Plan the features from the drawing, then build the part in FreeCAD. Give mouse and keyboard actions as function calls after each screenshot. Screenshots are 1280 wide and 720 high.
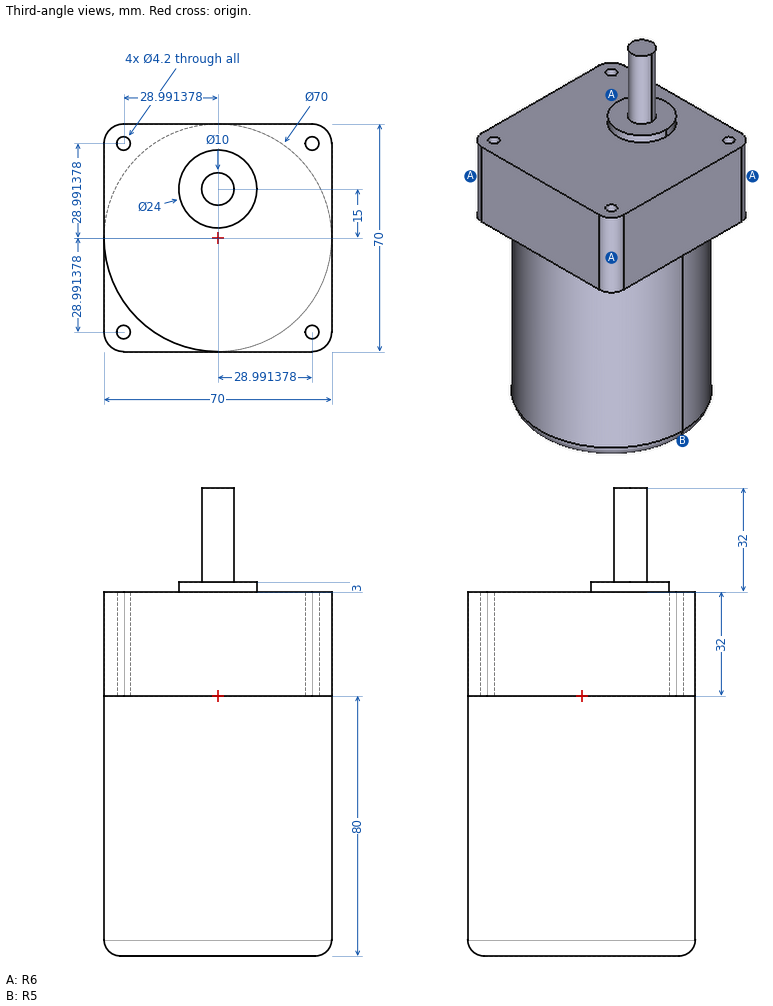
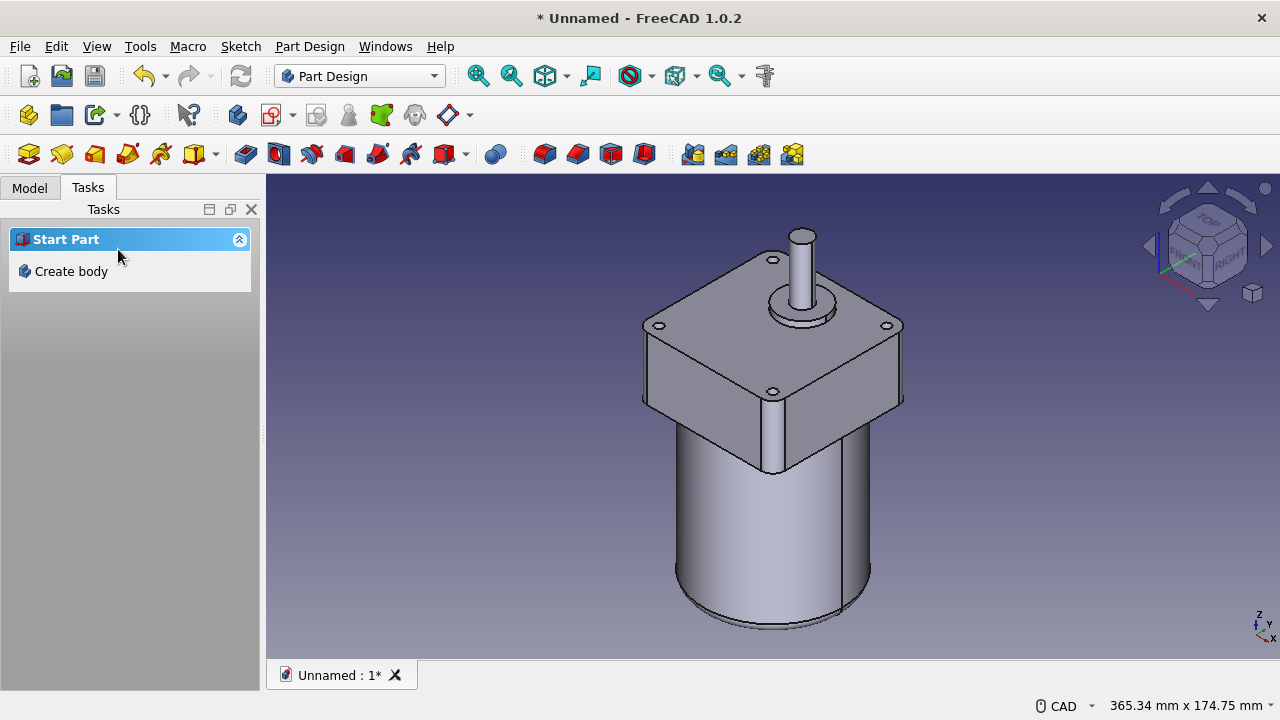
click(479, 76)